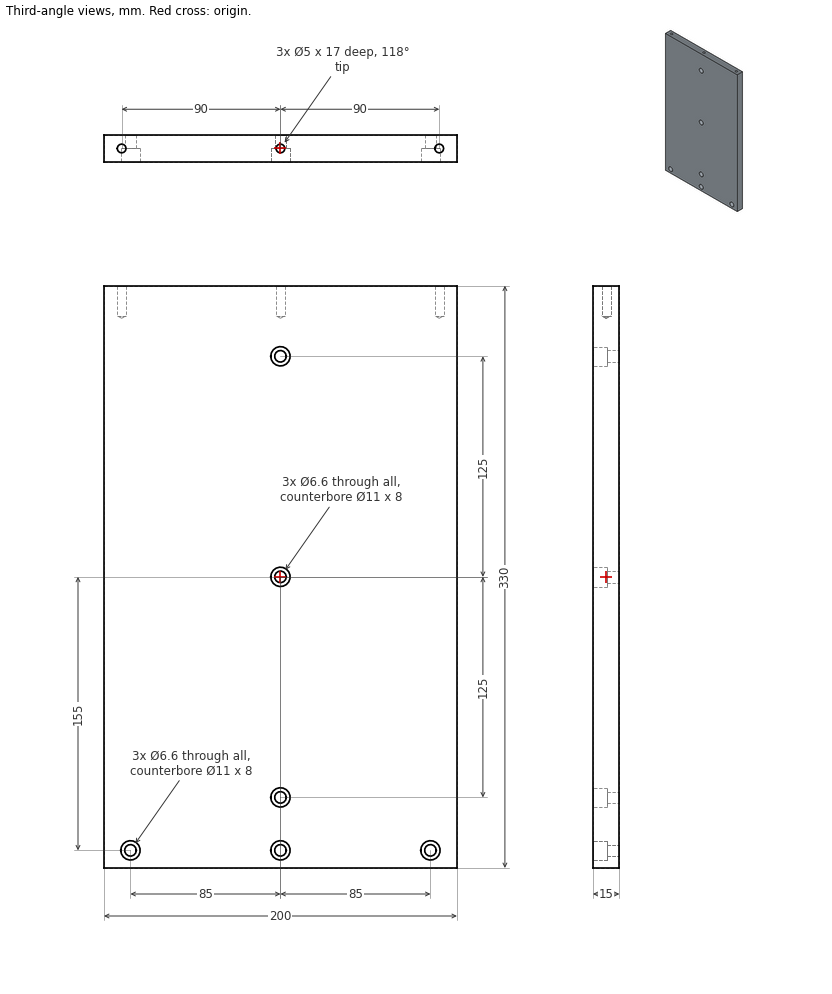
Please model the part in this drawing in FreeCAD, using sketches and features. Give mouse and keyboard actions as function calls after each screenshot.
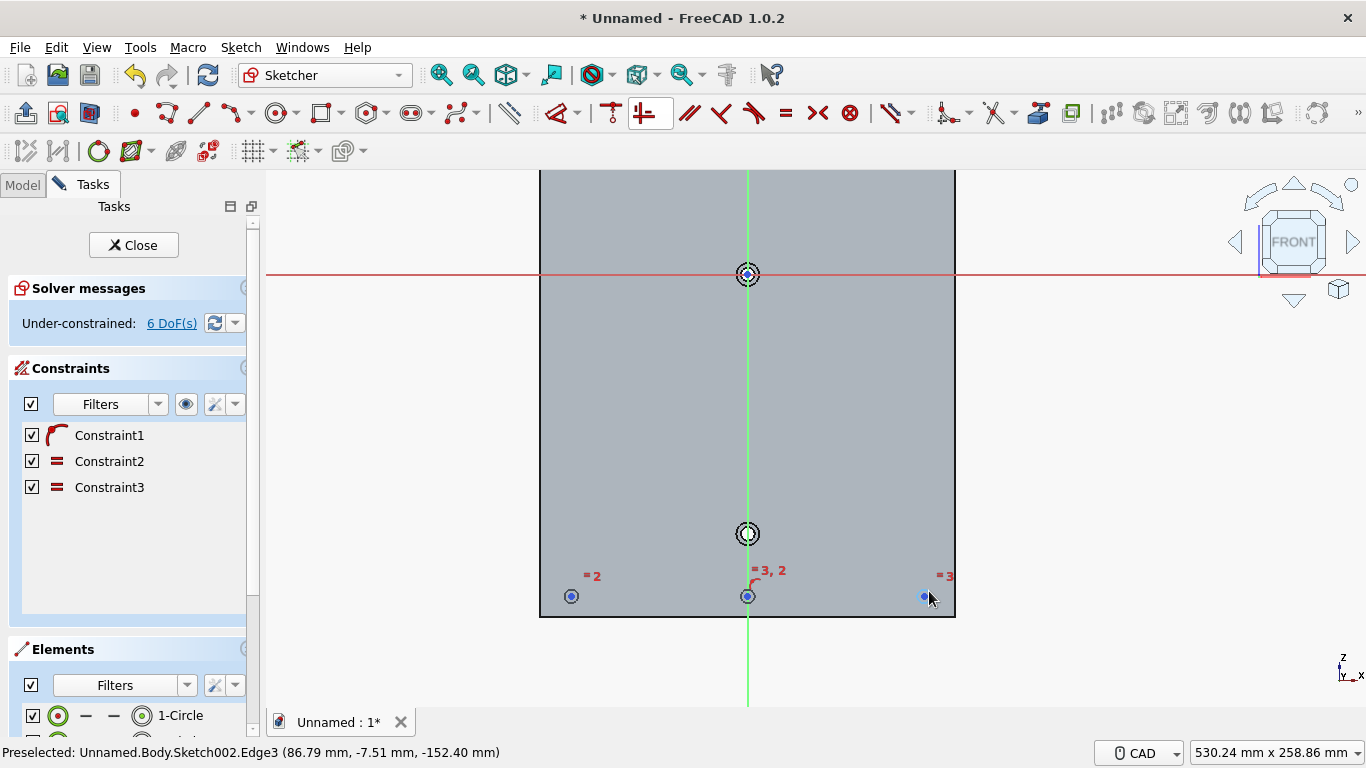
click(571, 596)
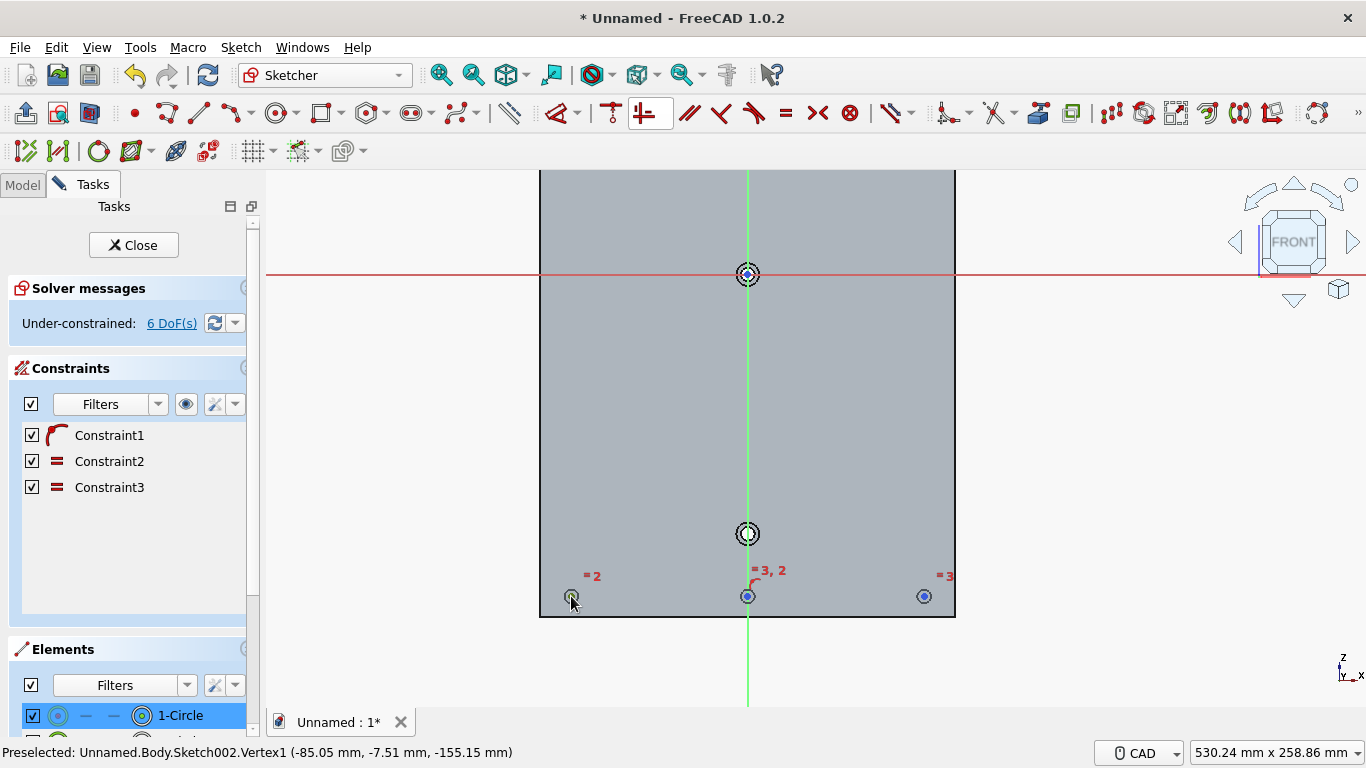
click(748, 596)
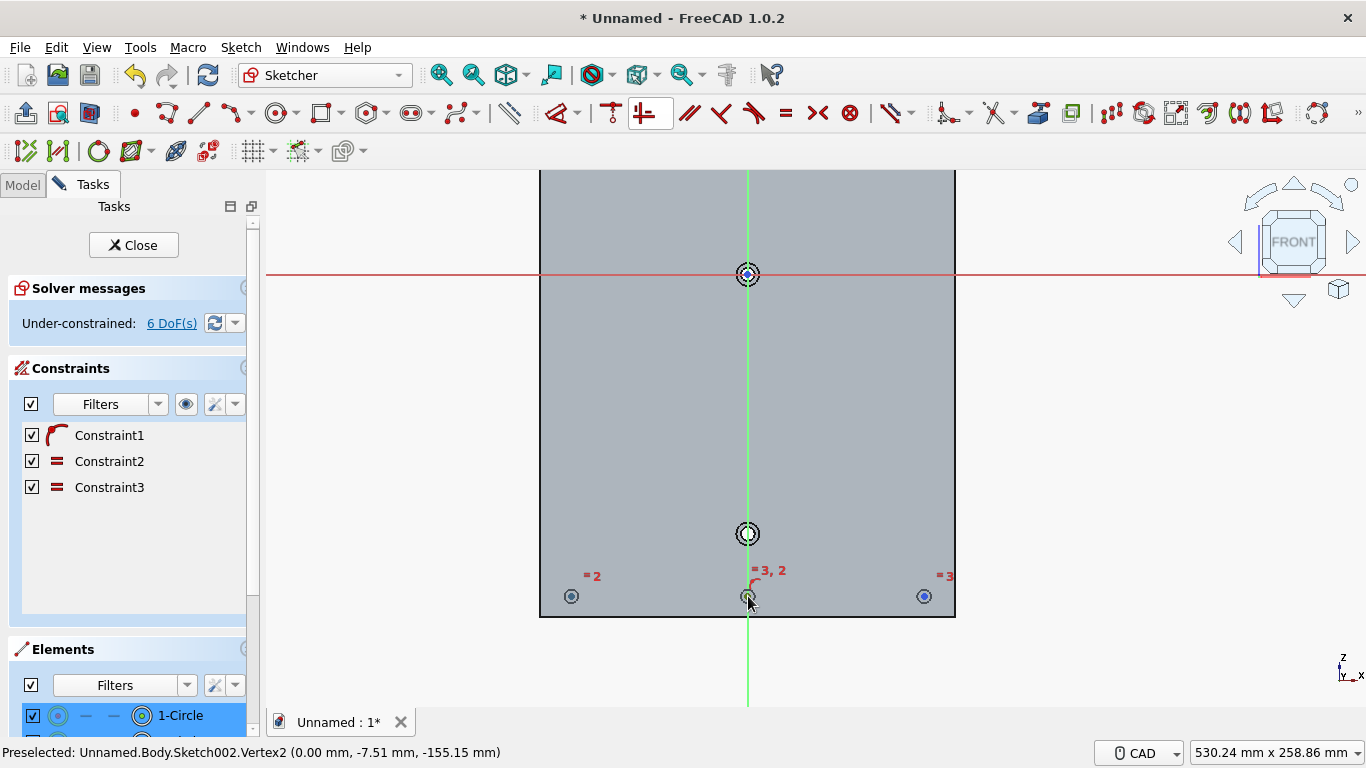
key(h)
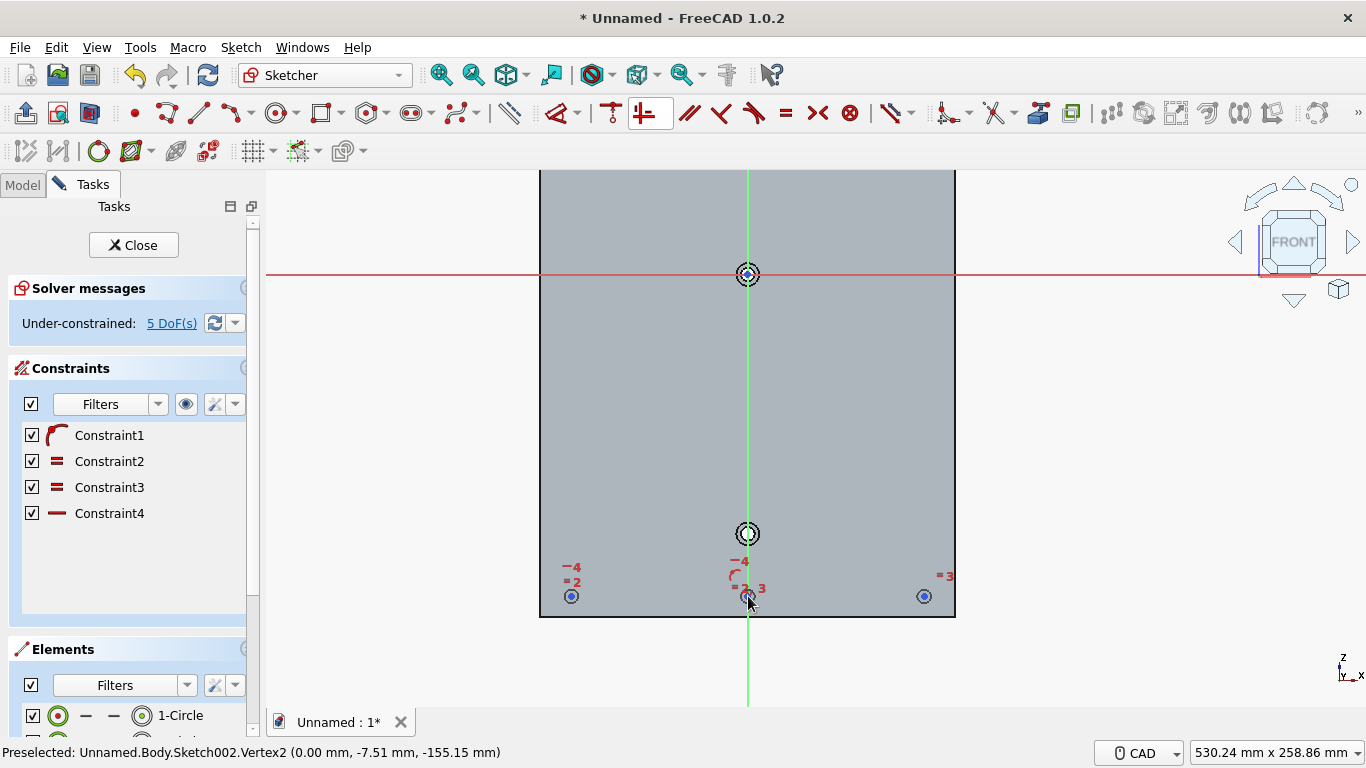
click(748, 596)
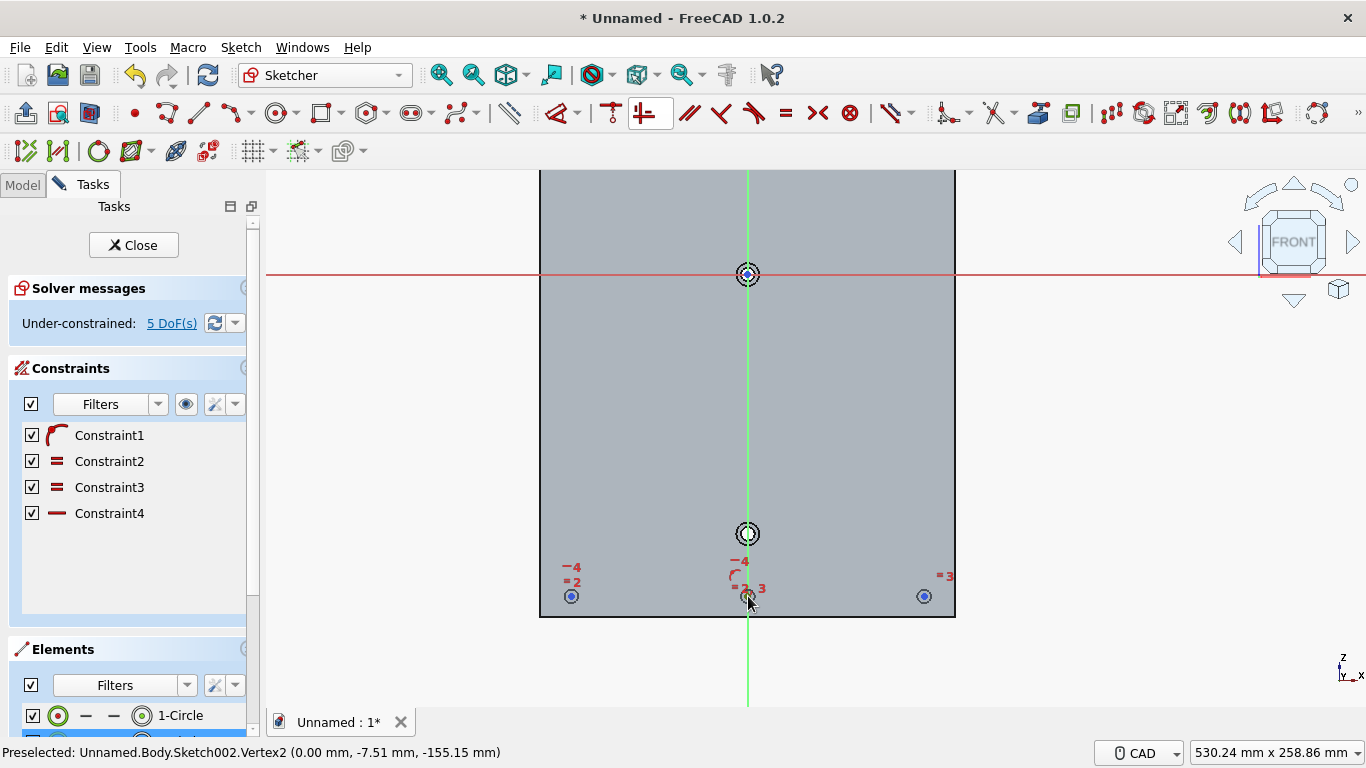
click(924, 596)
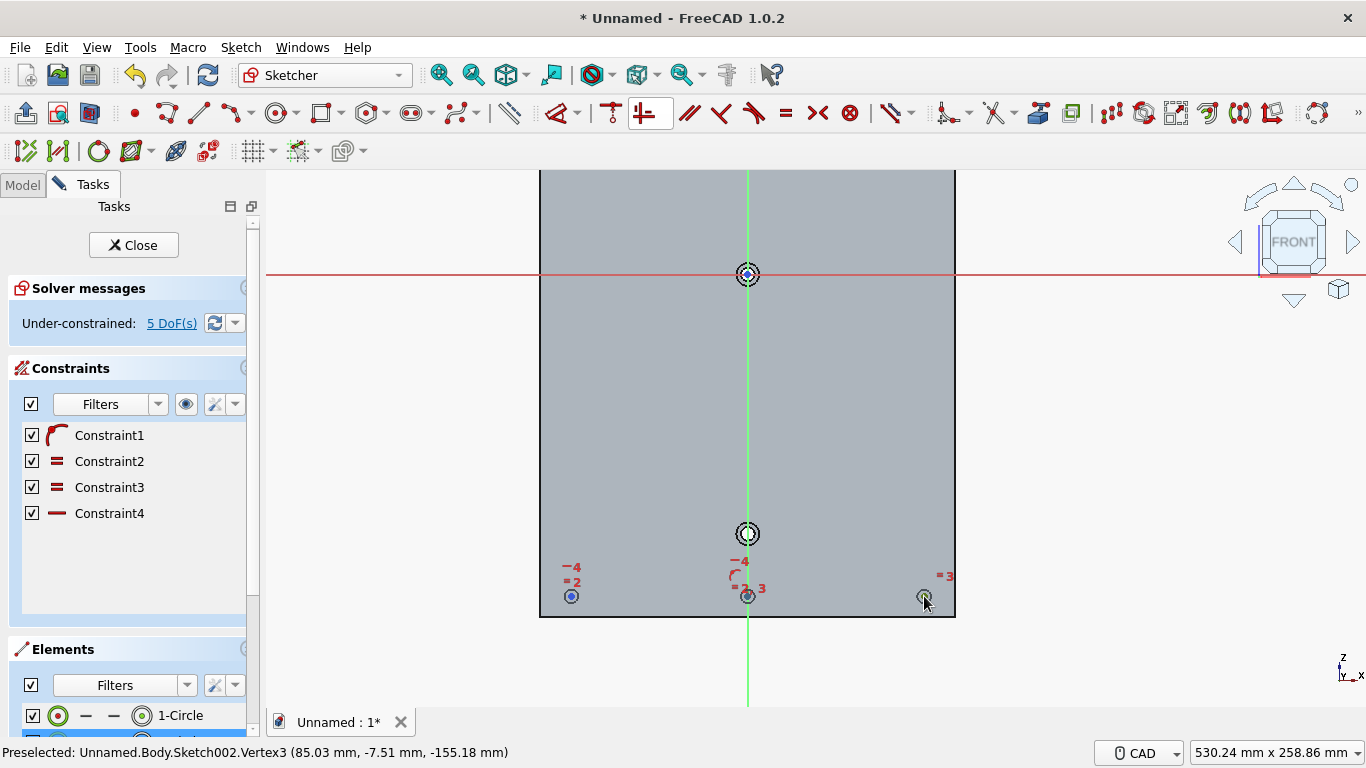
key(h)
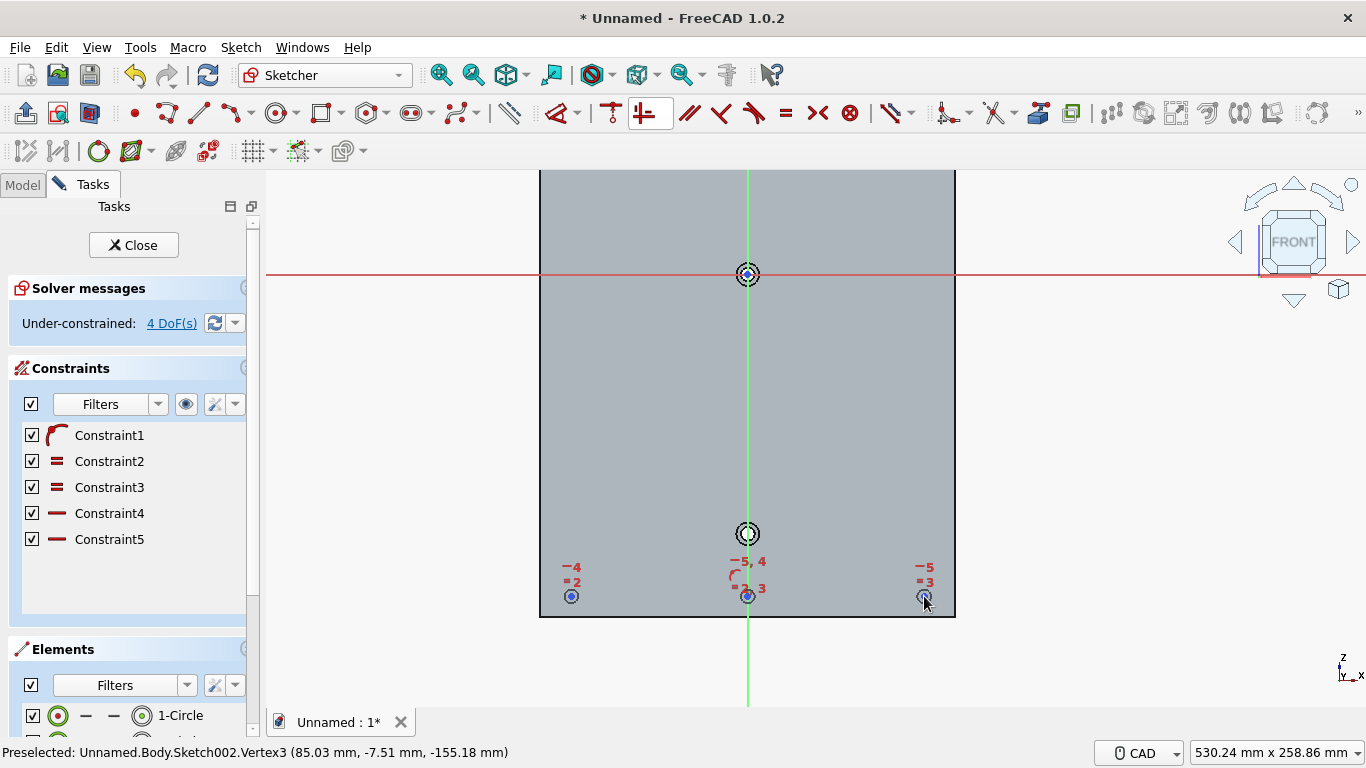
click(556, 114)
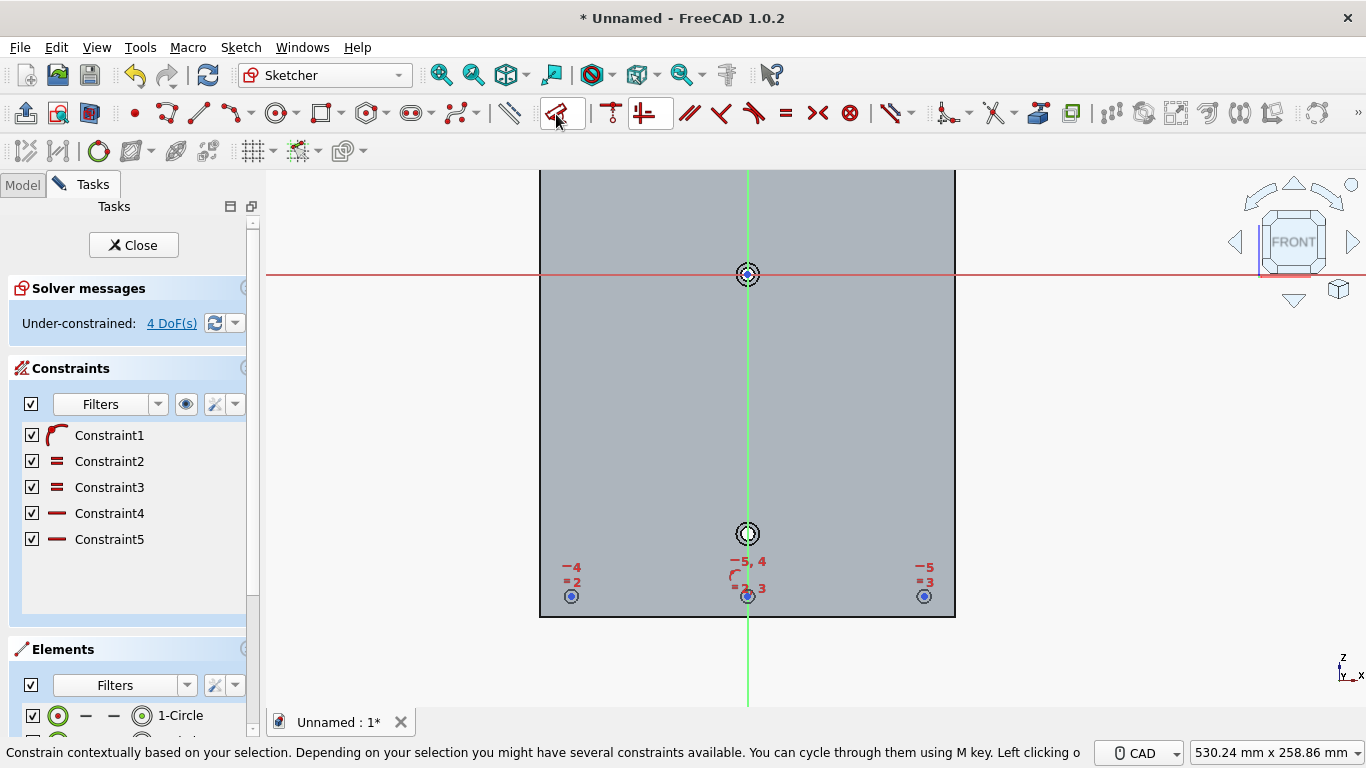
scroll(572, 590, up, 6)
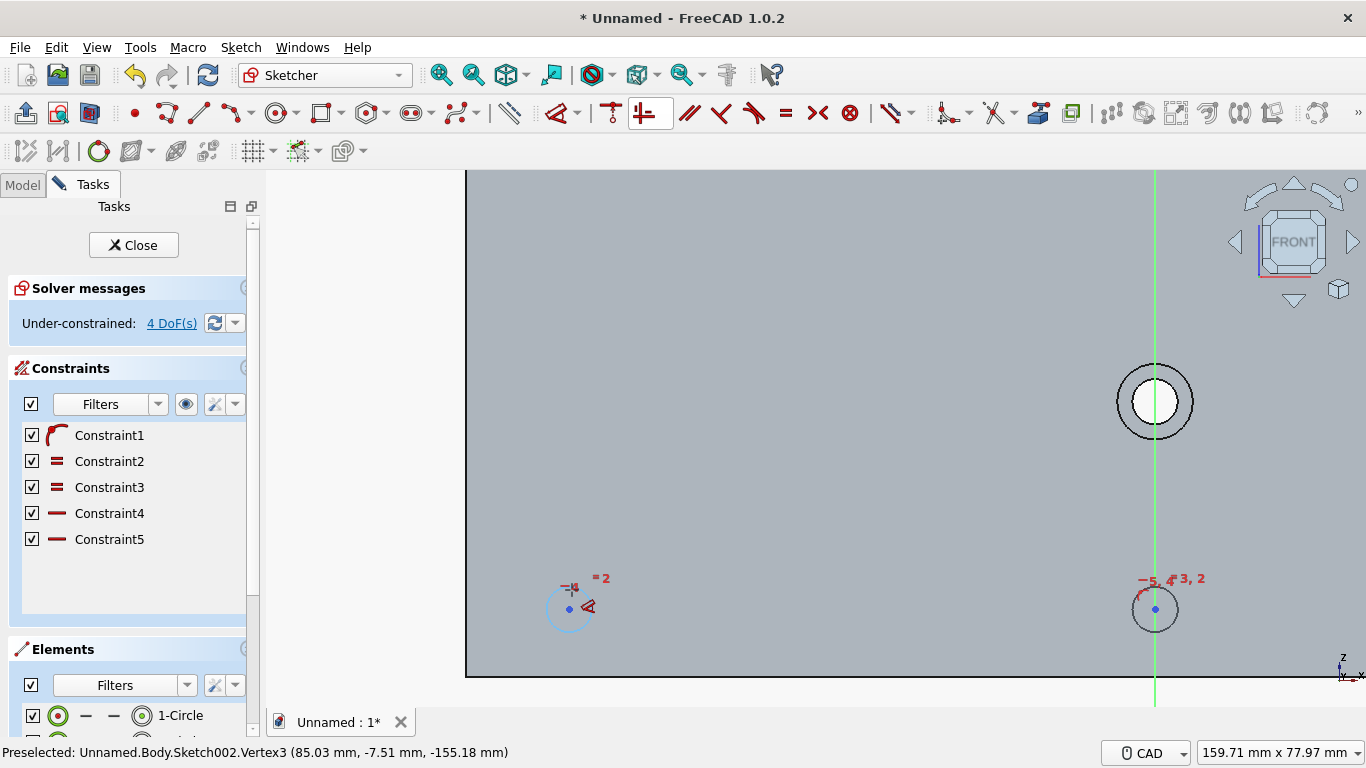
click(570, 587)
click(571, 555)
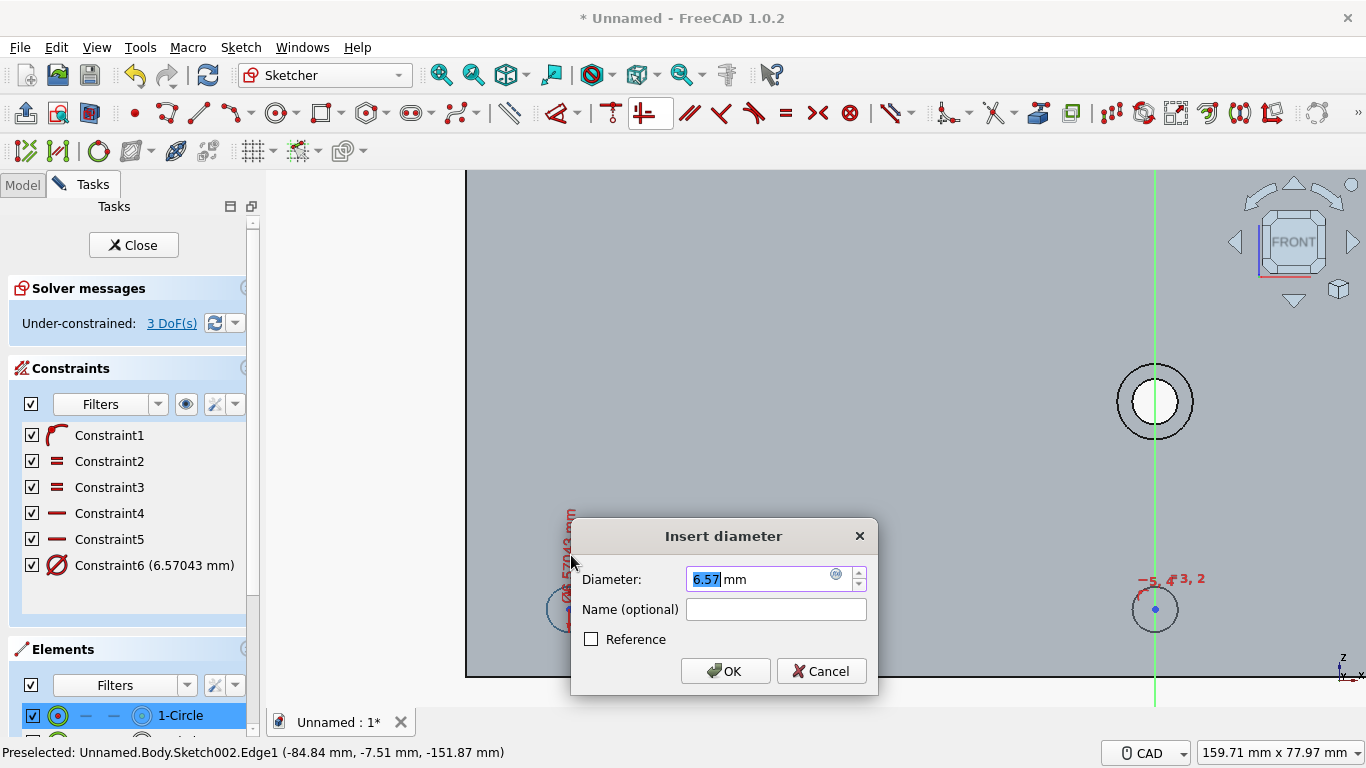
text(6.6)
key(Return)